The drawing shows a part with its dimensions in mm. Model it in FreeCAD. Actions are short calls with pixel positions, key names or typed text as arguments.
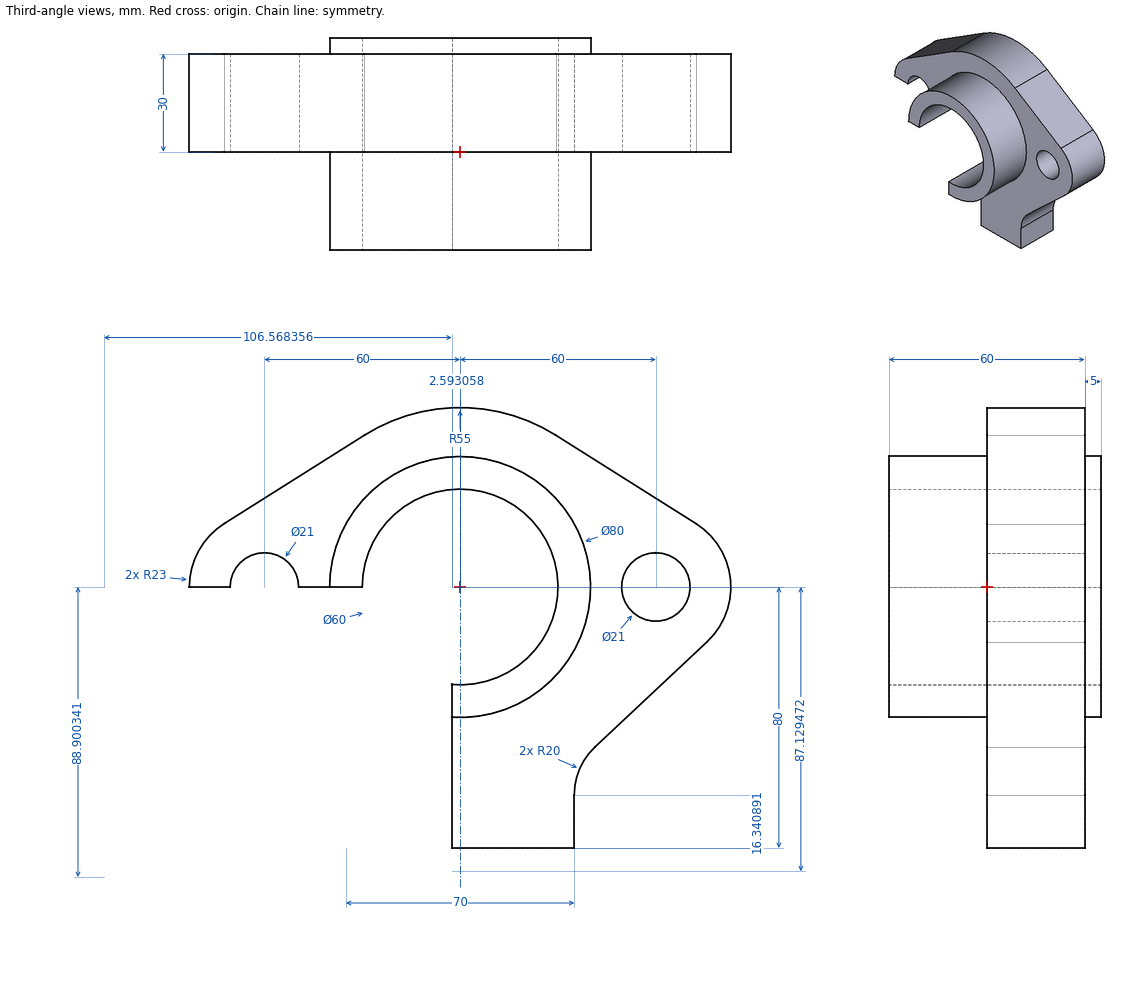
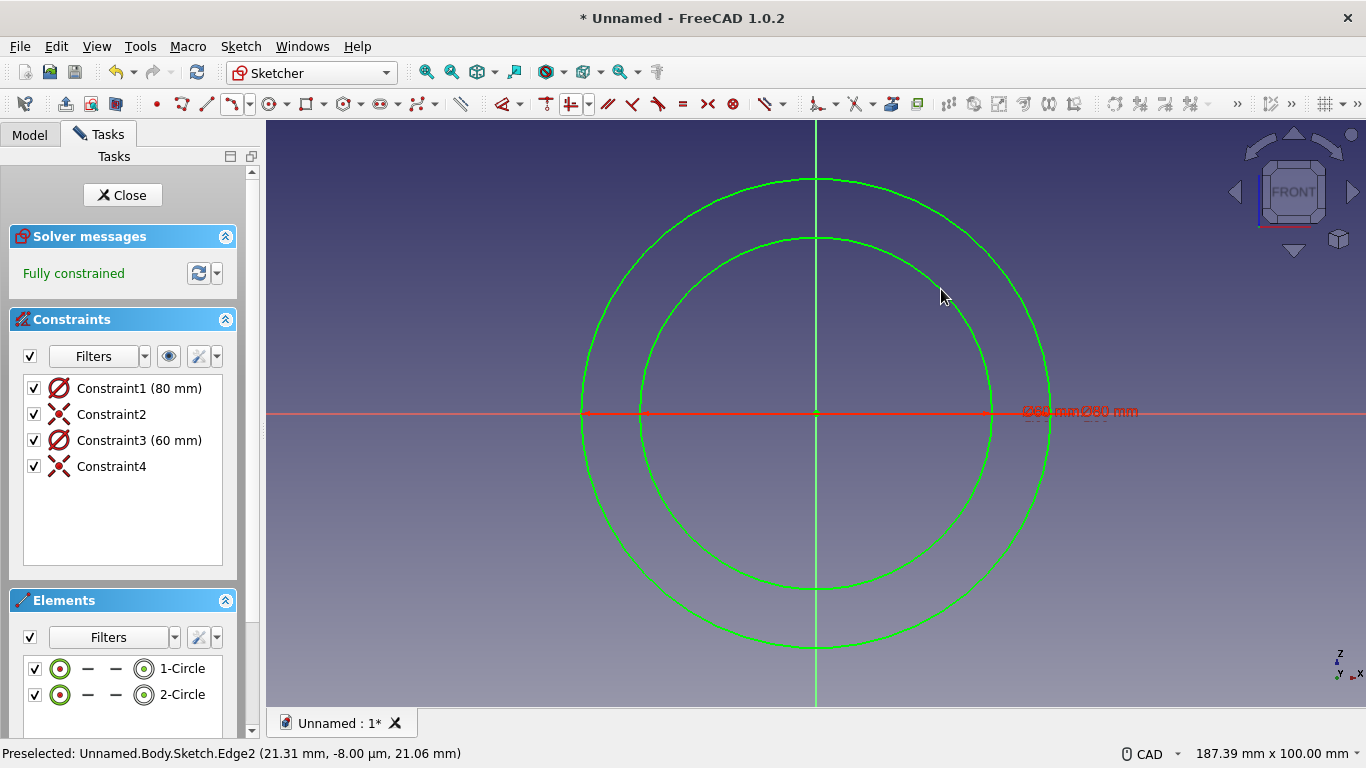
click(123, 195)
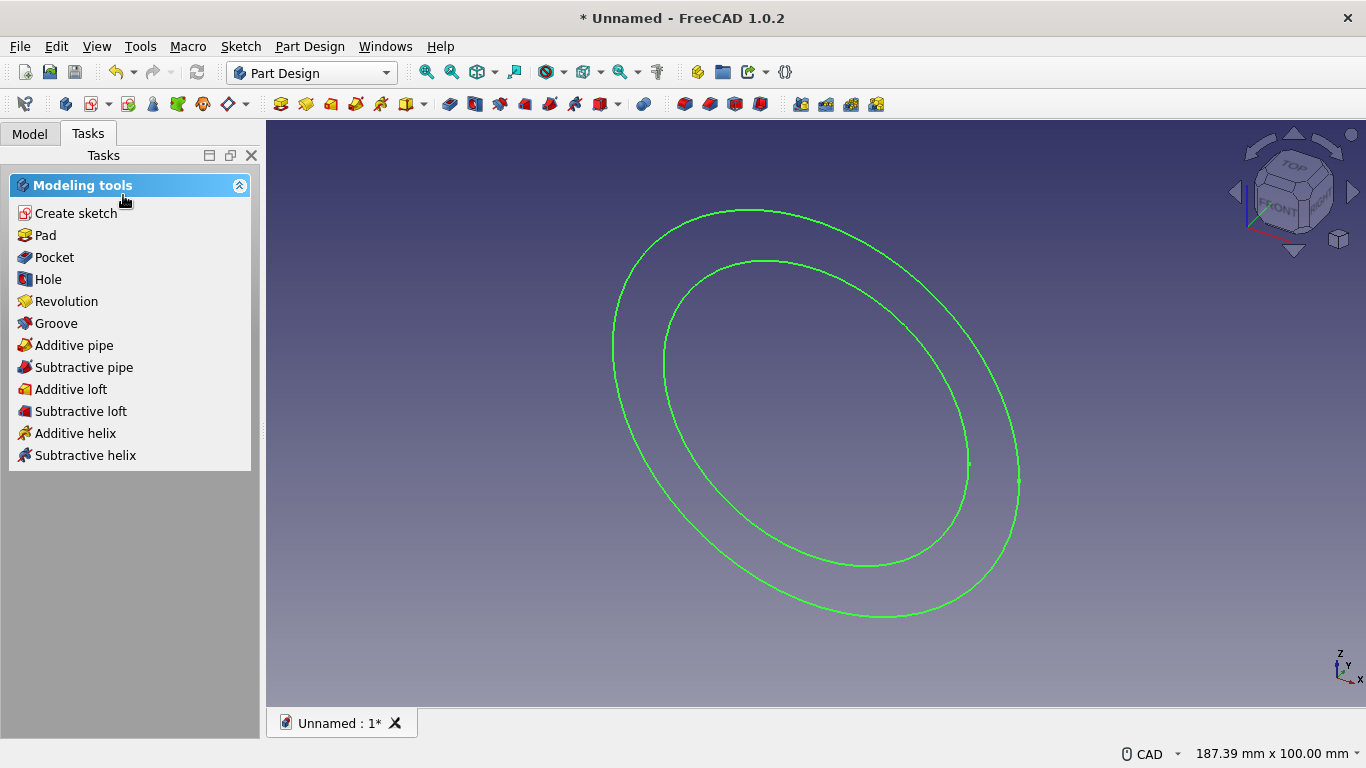
click(281, 104)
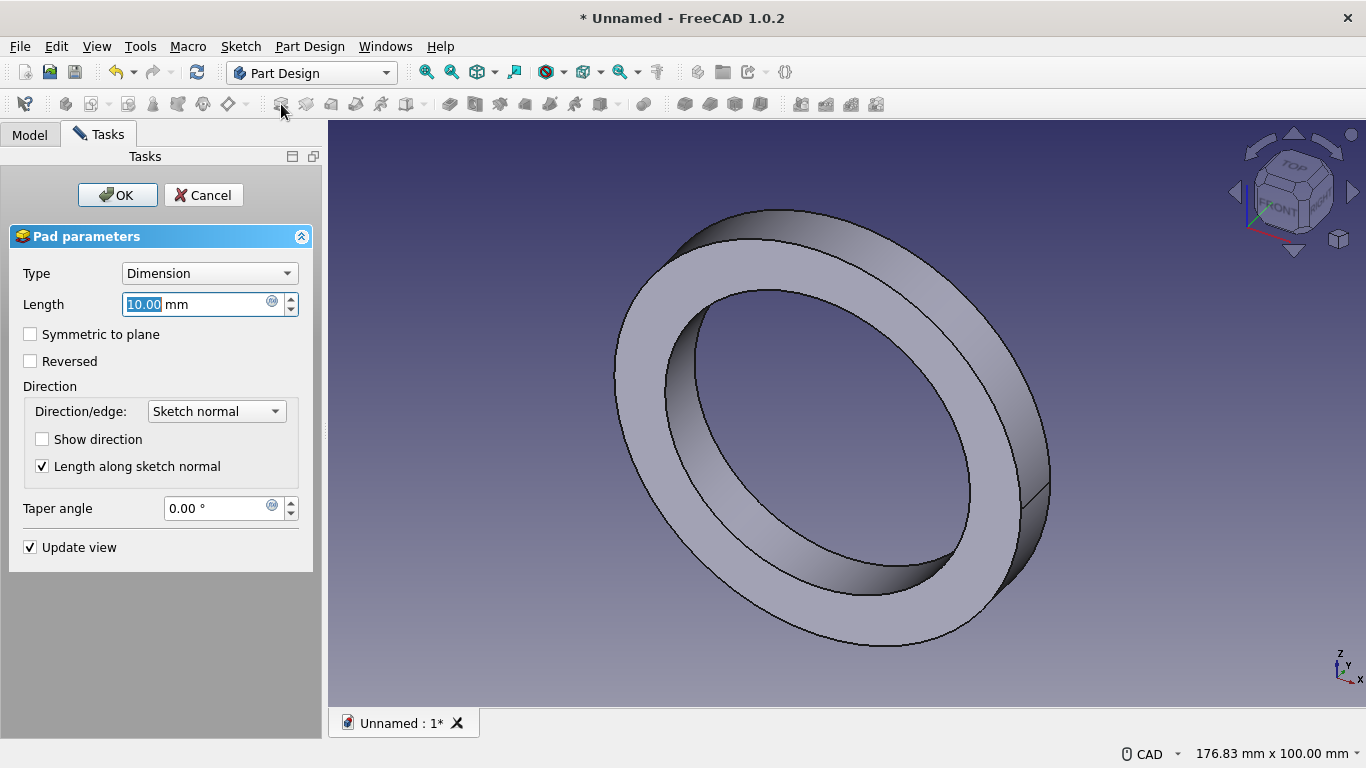
text(60)
key(Tab)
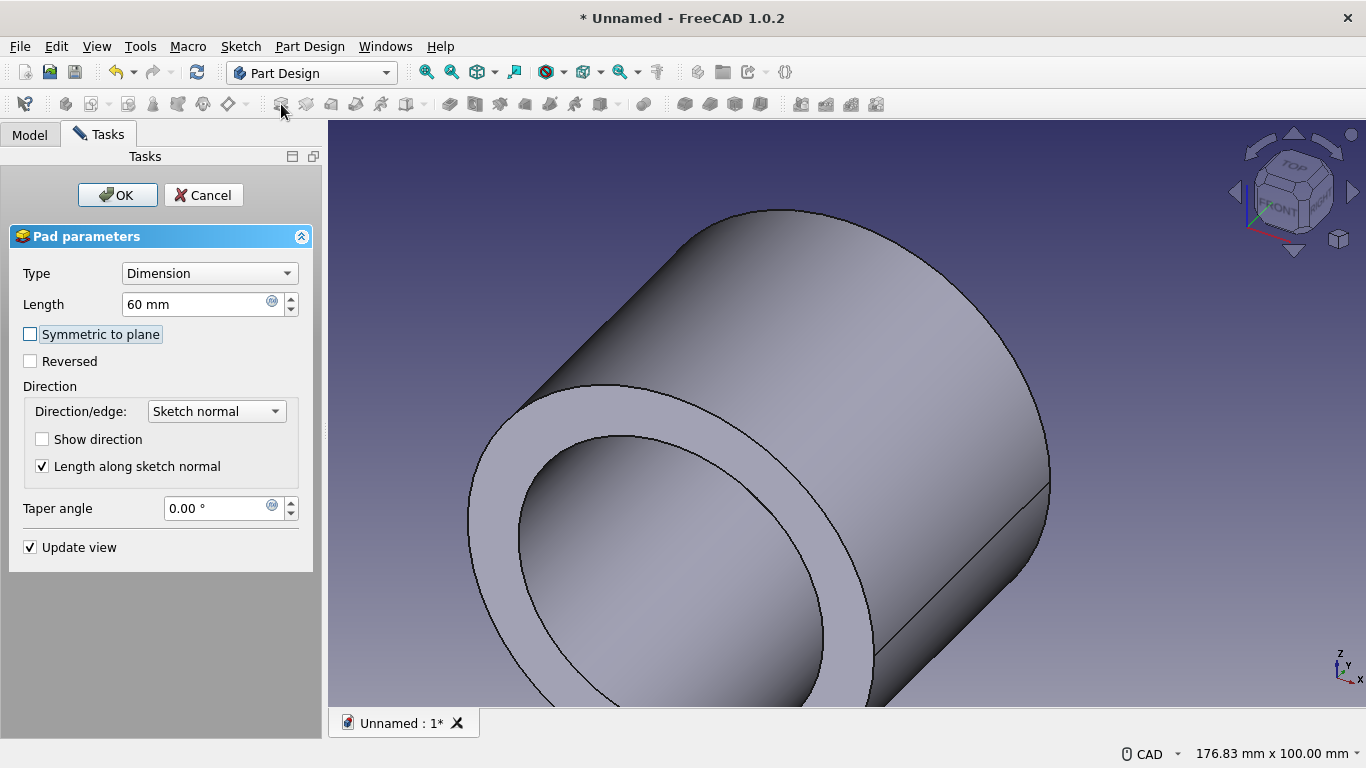
click(31, 334)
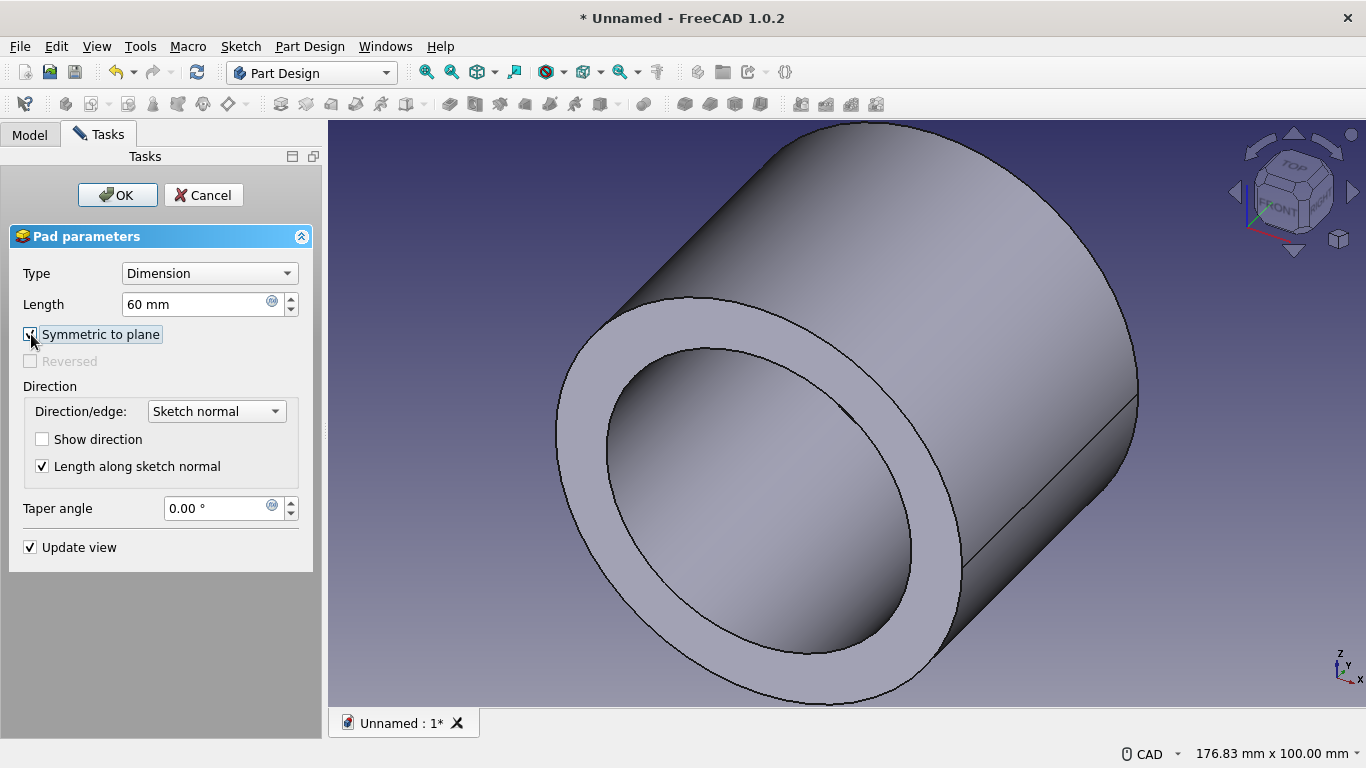
click(118, 195)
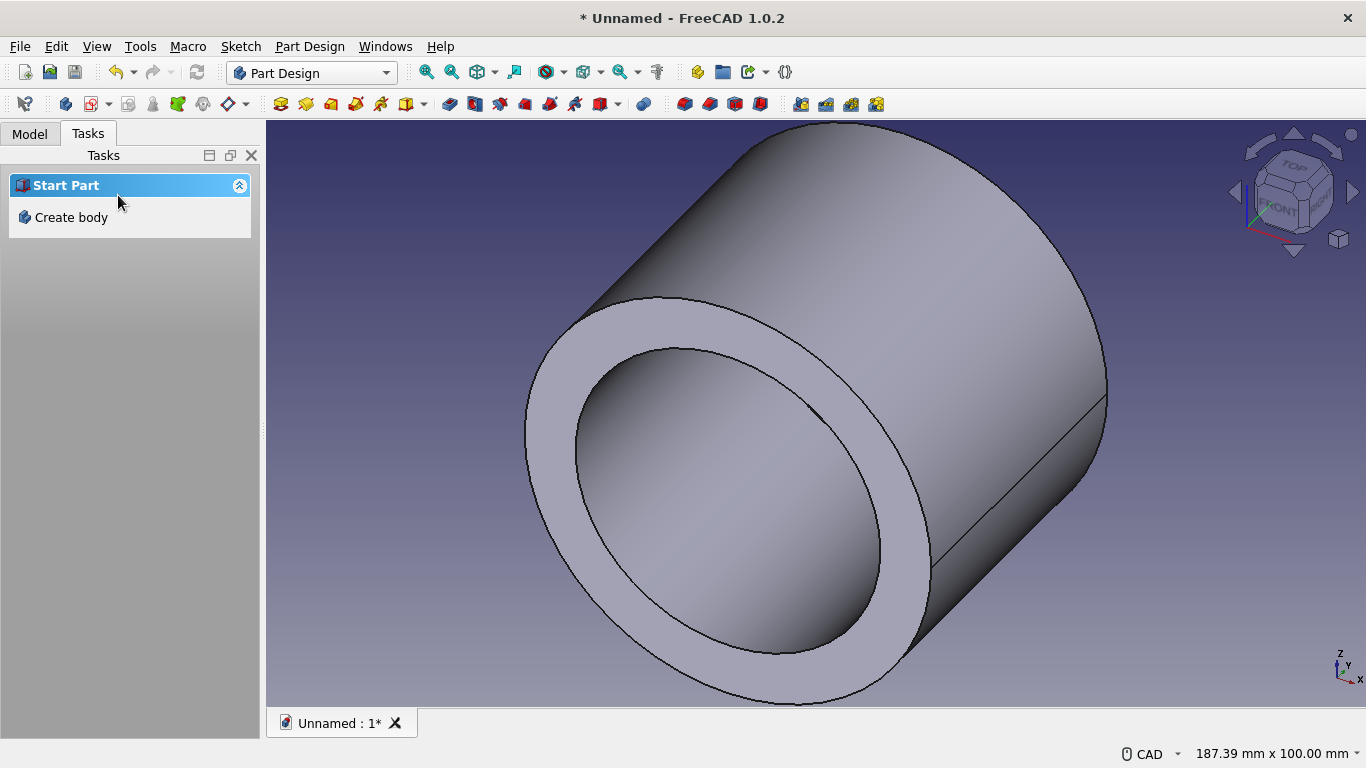
click(427, 72)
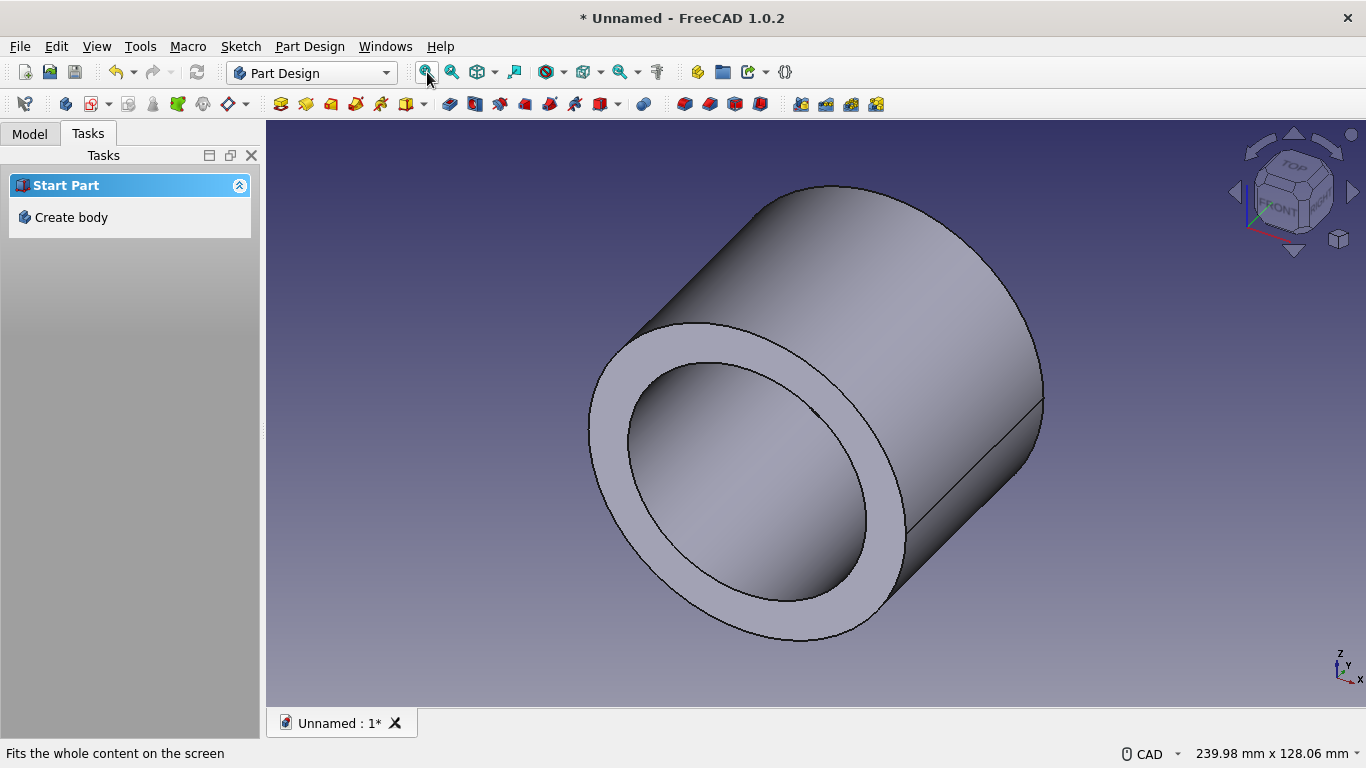
key(4)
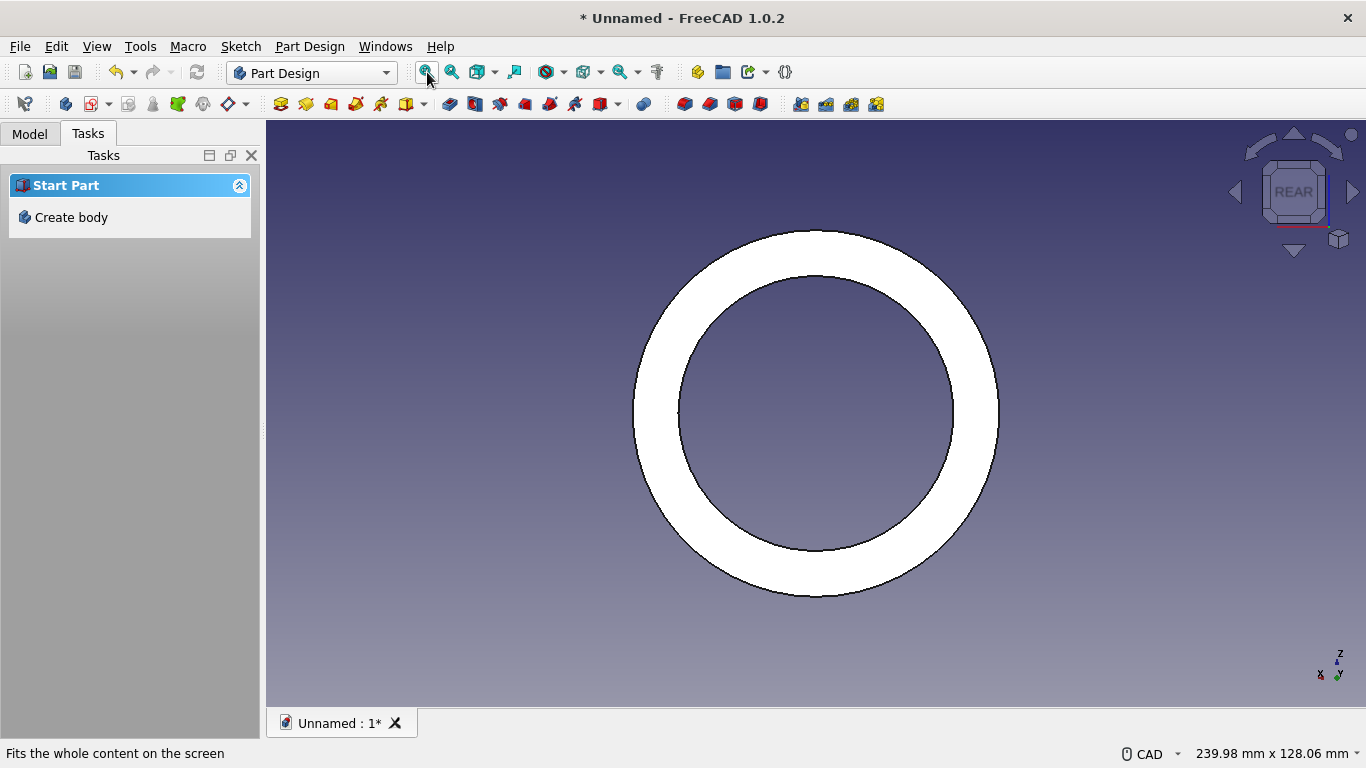
click(659, 412)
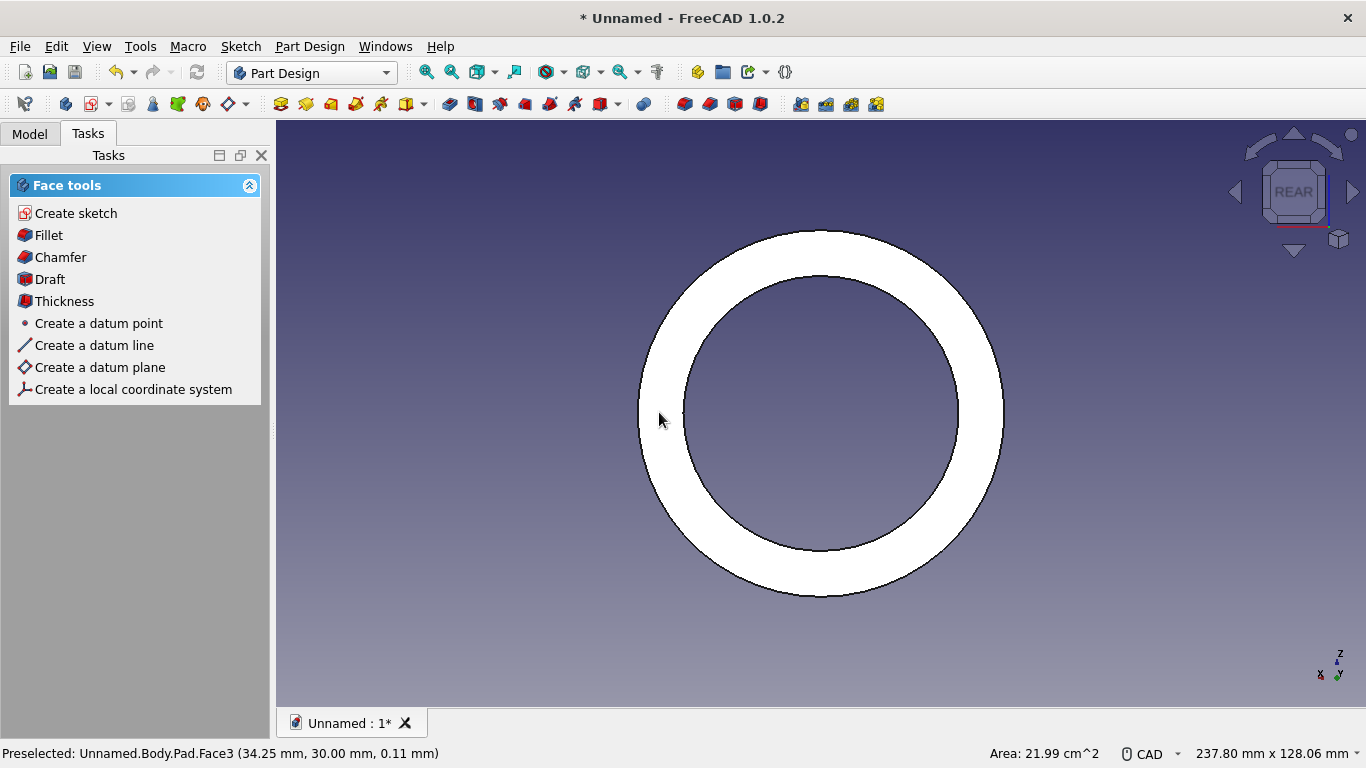
click(90, 104)